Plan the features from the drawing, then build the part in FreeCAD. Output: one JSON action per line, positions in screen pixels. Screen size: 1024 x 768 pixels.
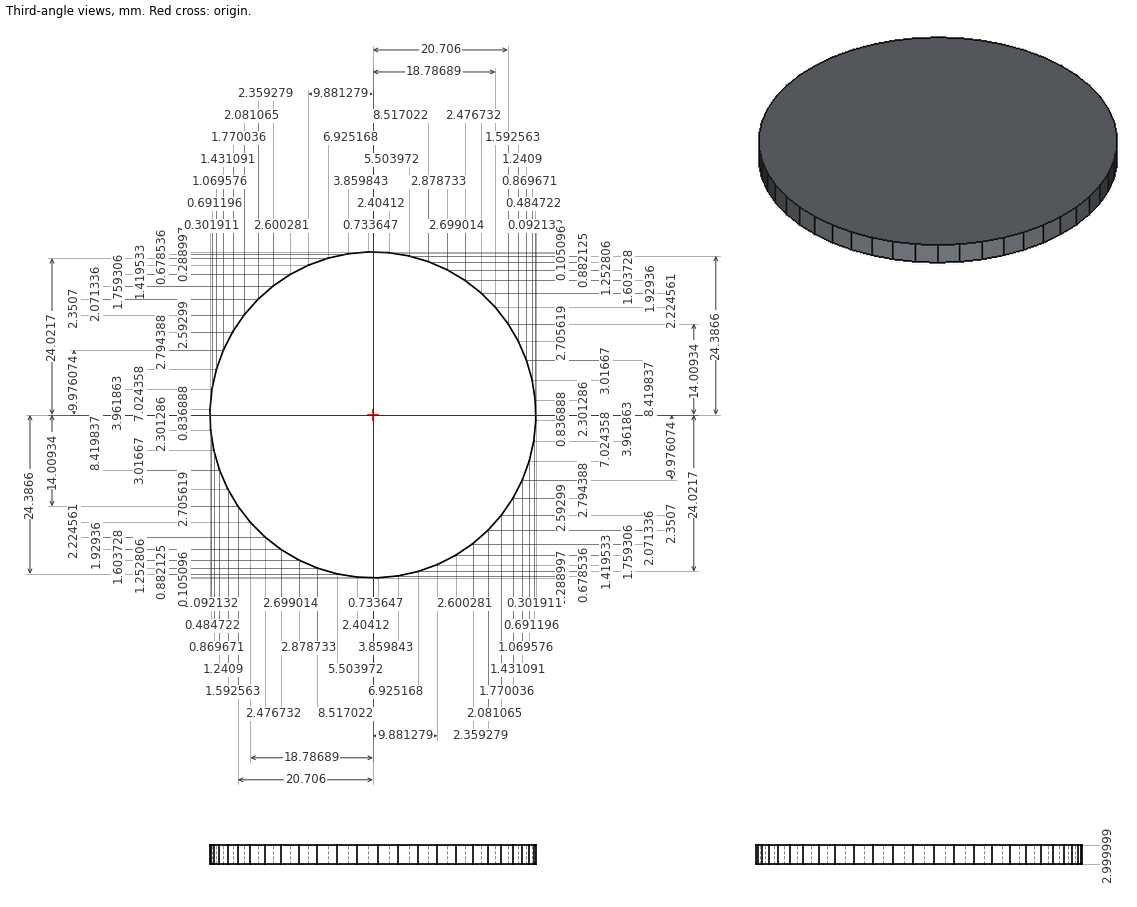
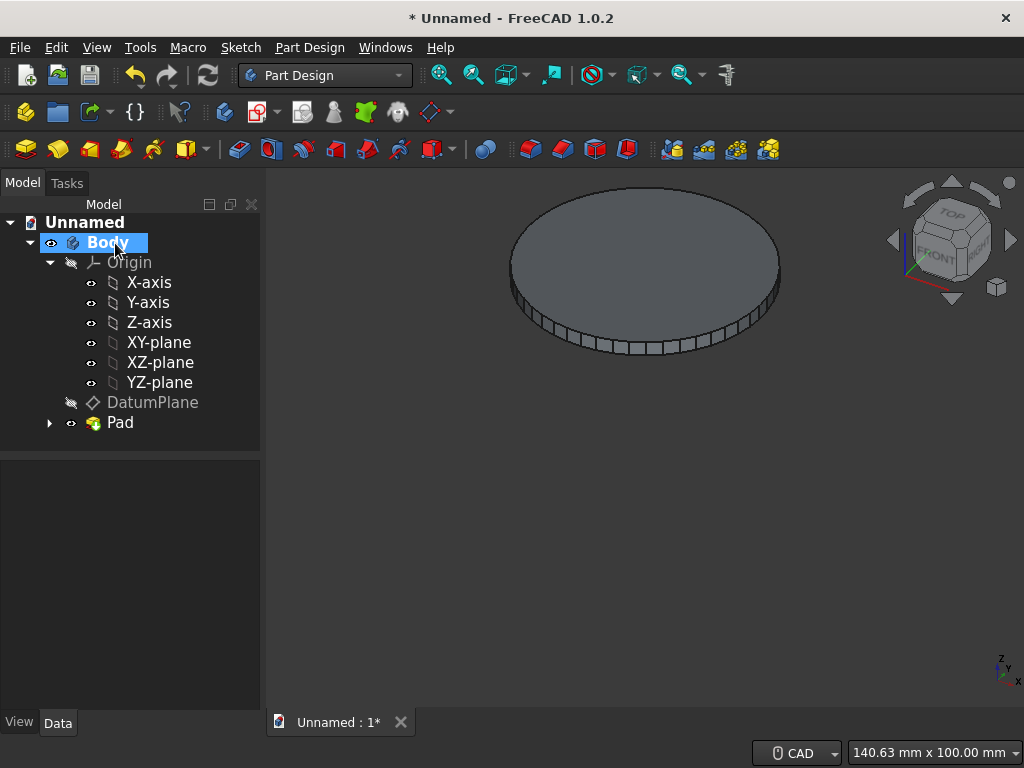
{"action": "key", "text": "0"}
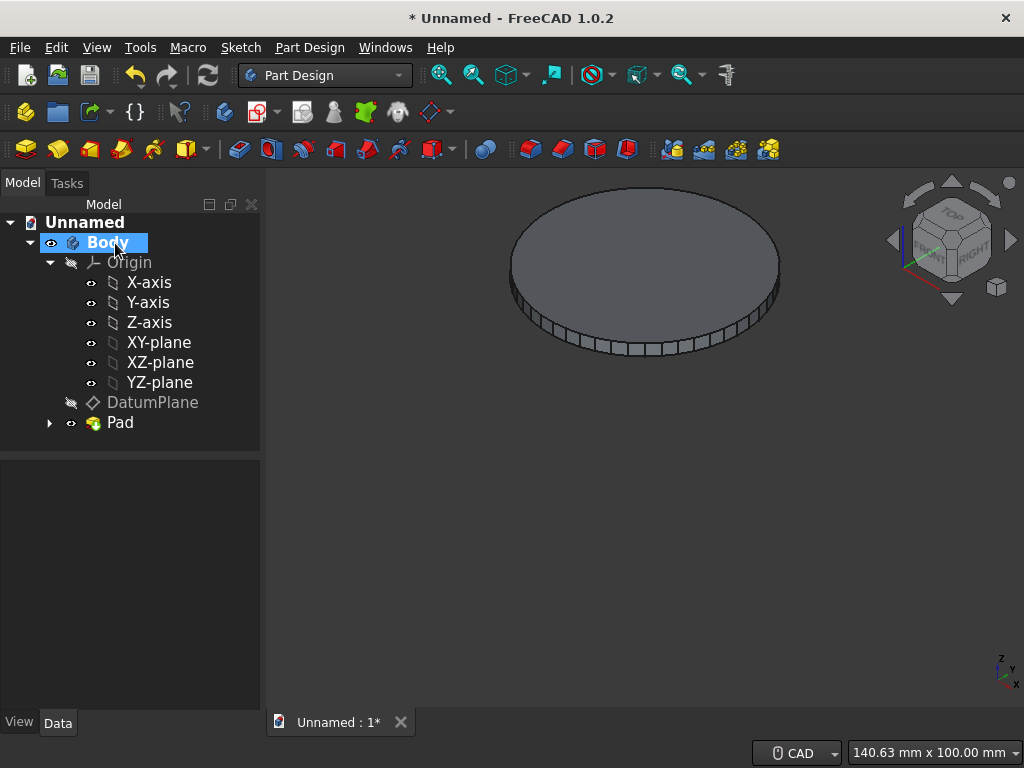
{"action": "left_click", "coordinate": [442, 76]}